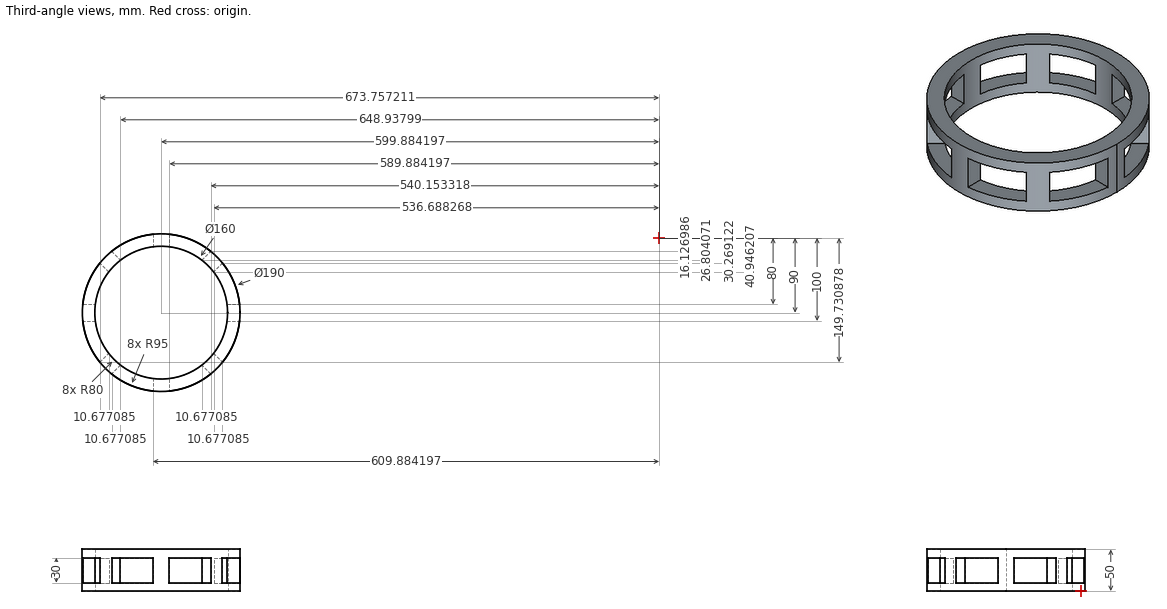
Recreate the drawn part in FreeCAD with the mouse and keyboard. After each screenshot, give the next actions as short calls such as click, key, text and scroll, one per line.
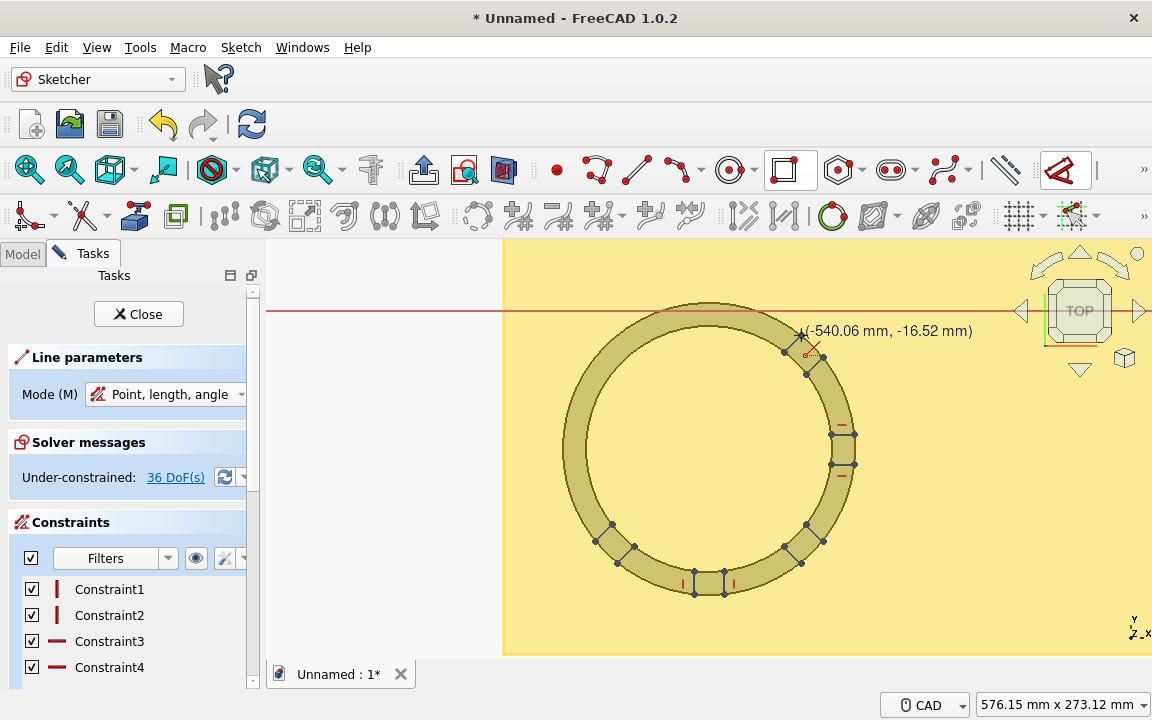
scroll(724, 304, up, 5)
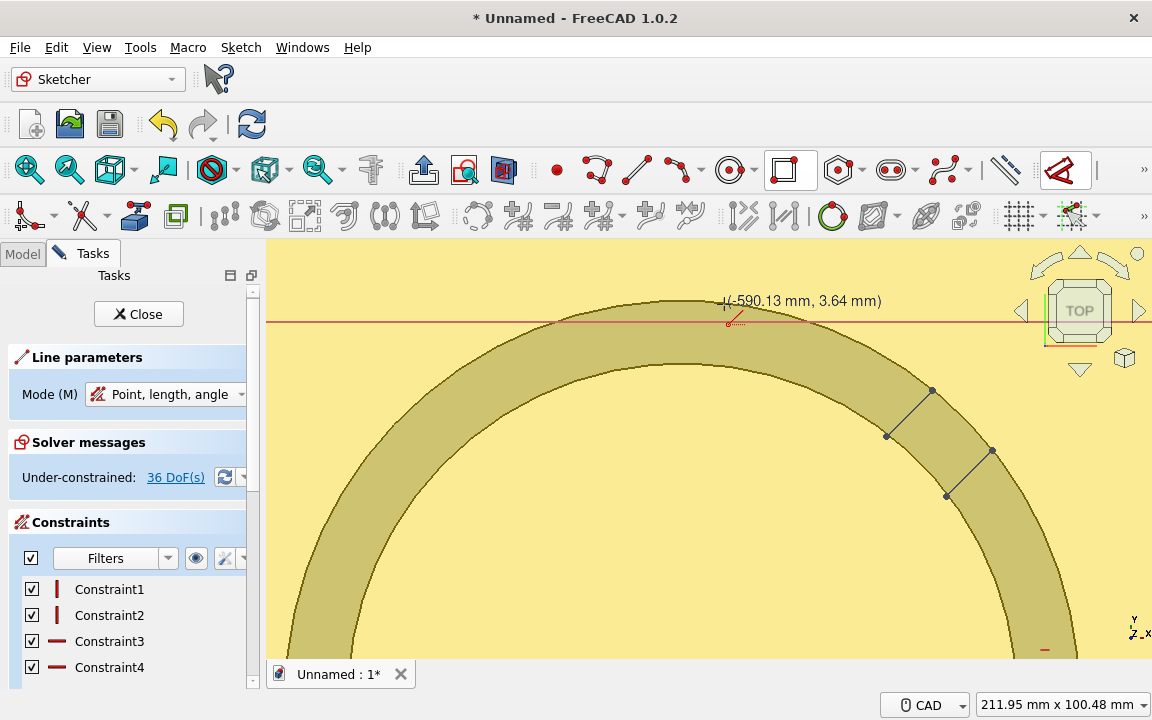
click(724, 303)
click(724, 366)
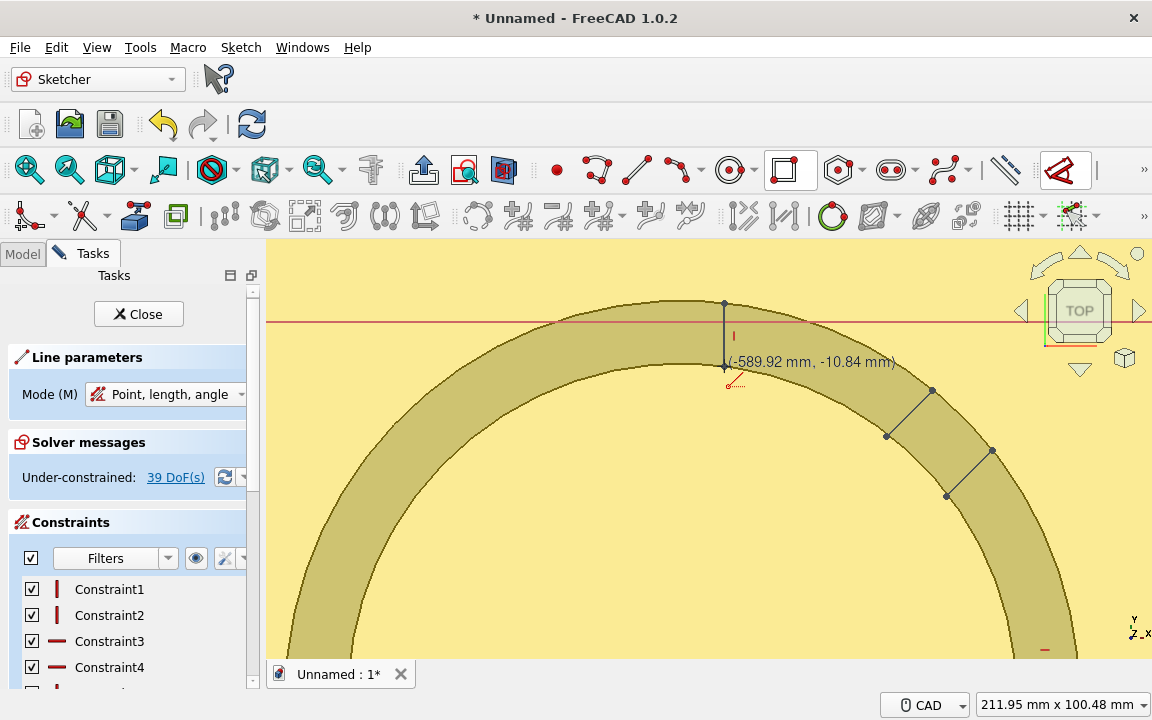
click(641, 366)
click(641, 303)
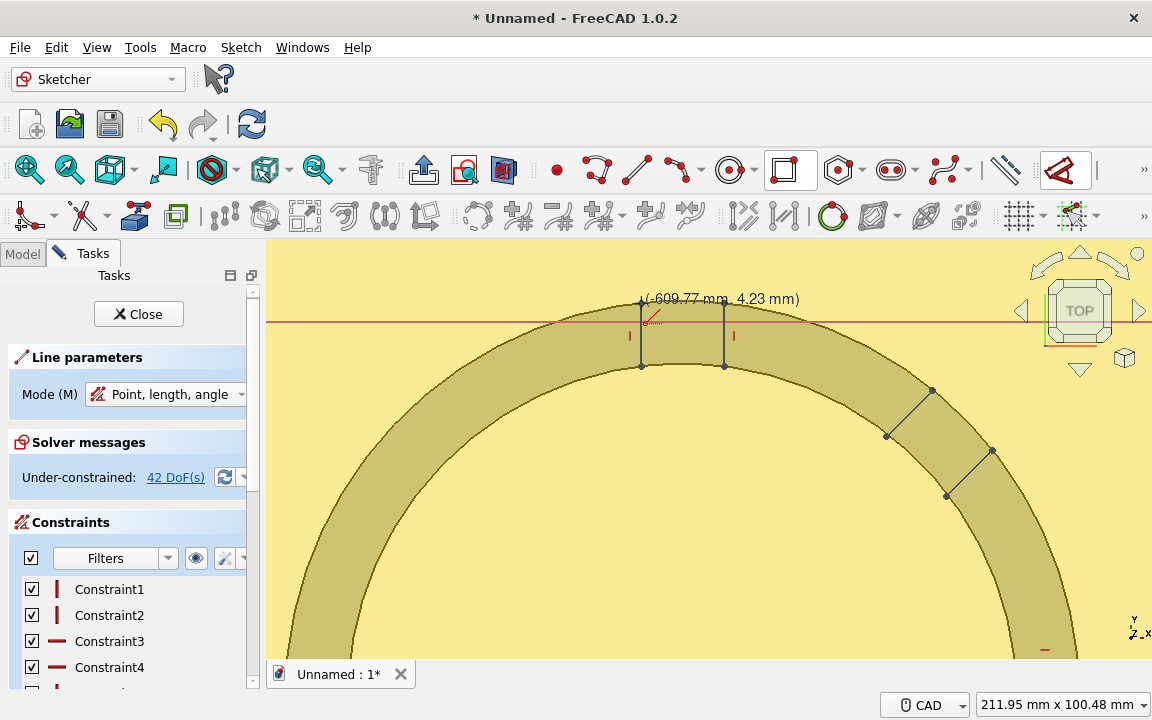
click(433, 389)
click(477, 434)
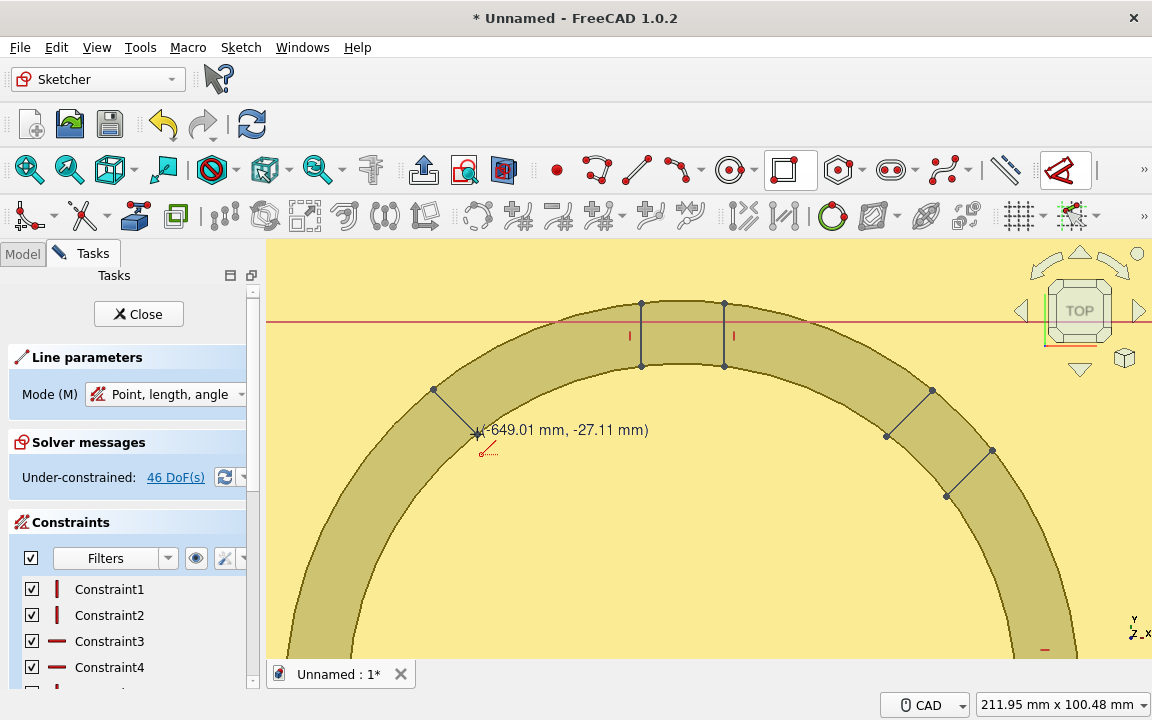
click(418, 493)
click(374, 448)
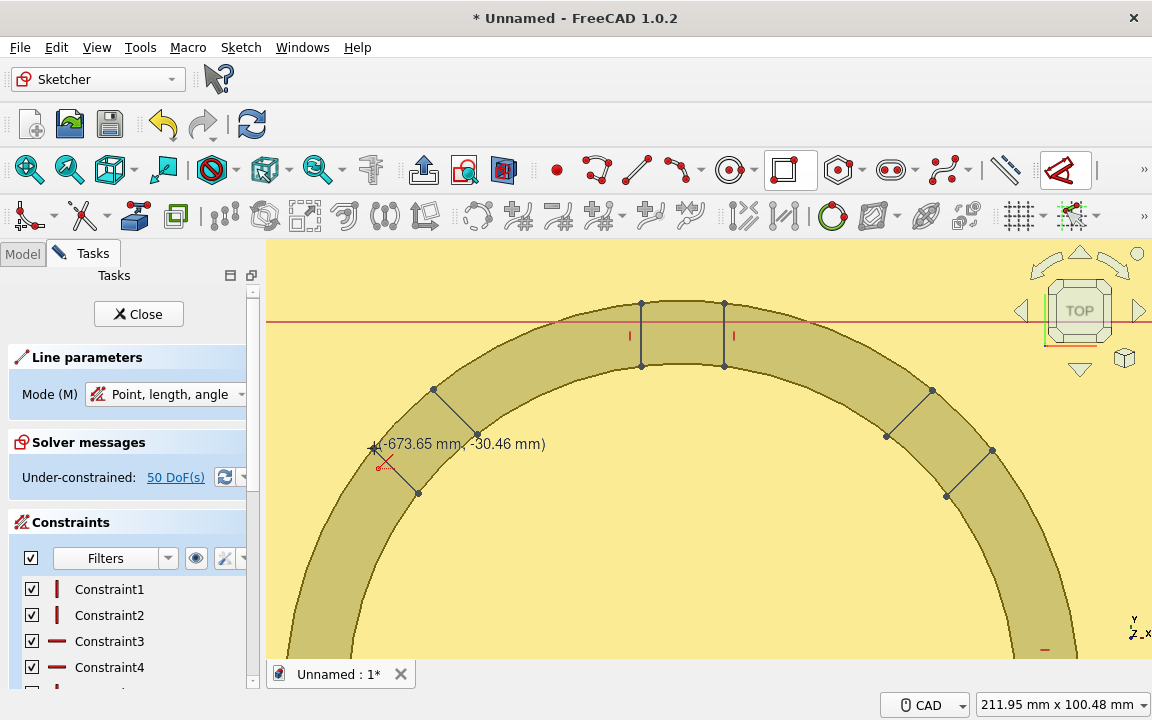
scroll(622, 342, down, 6)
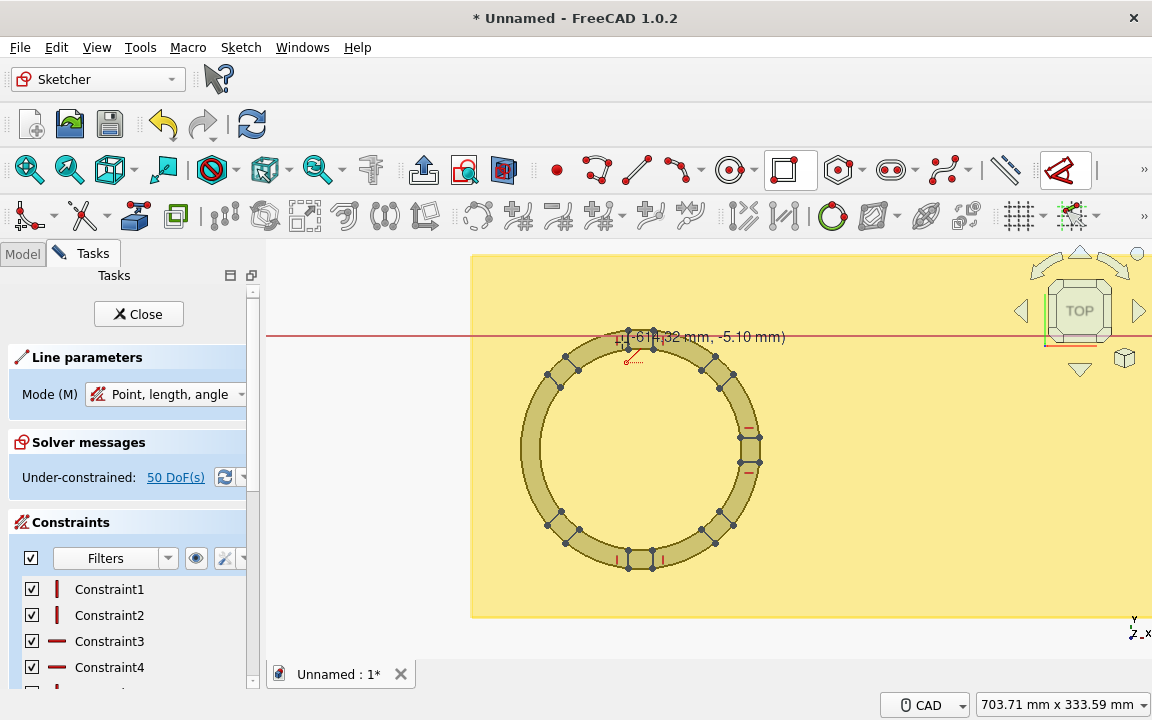
click(522, 437)
click(541, 437)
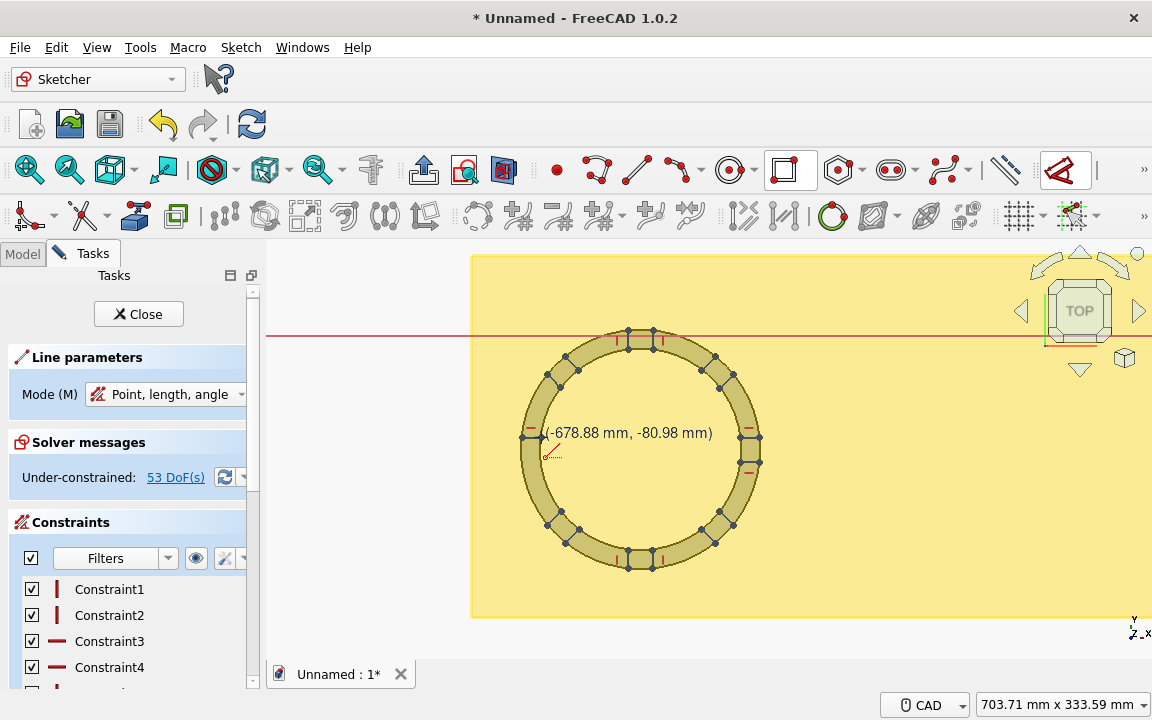
click(541, 462)
click(522, 462)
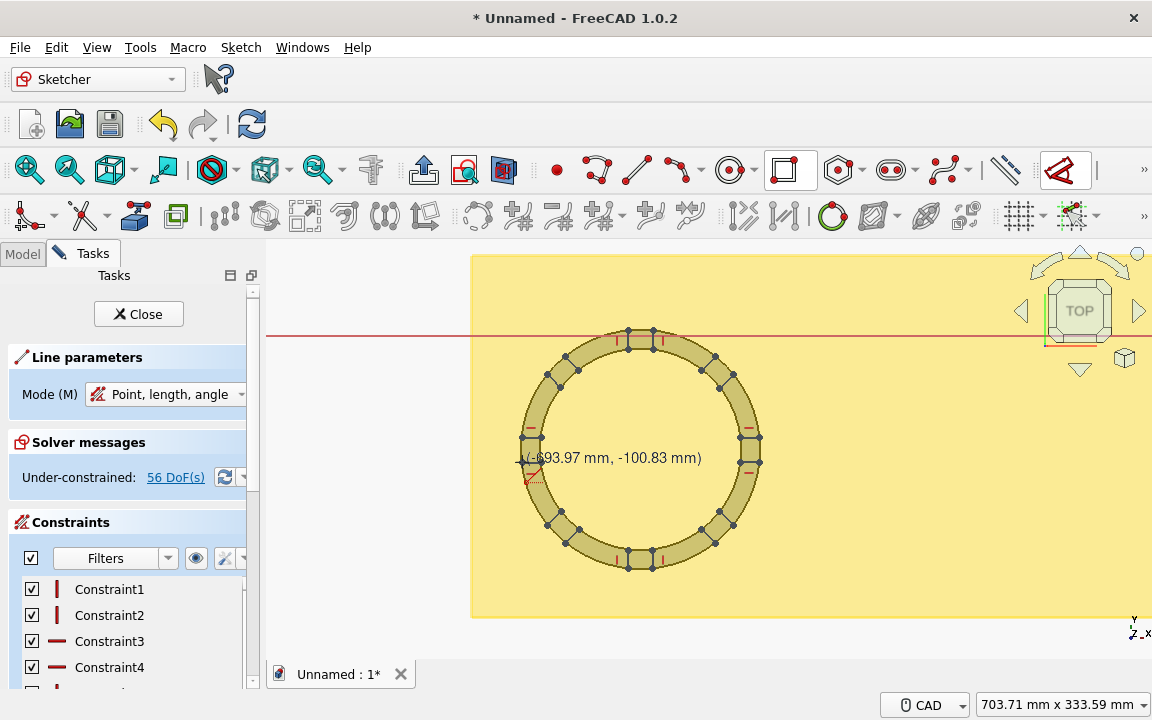
click(678, 170)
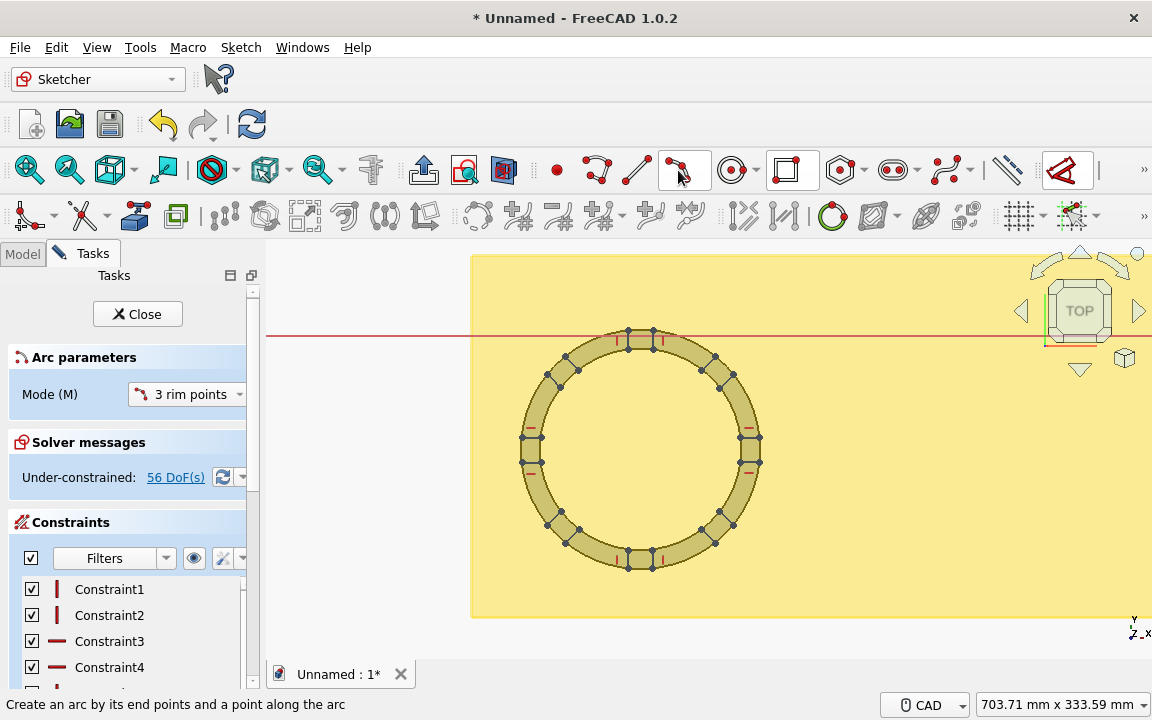
scroll(561, 511, up, 3)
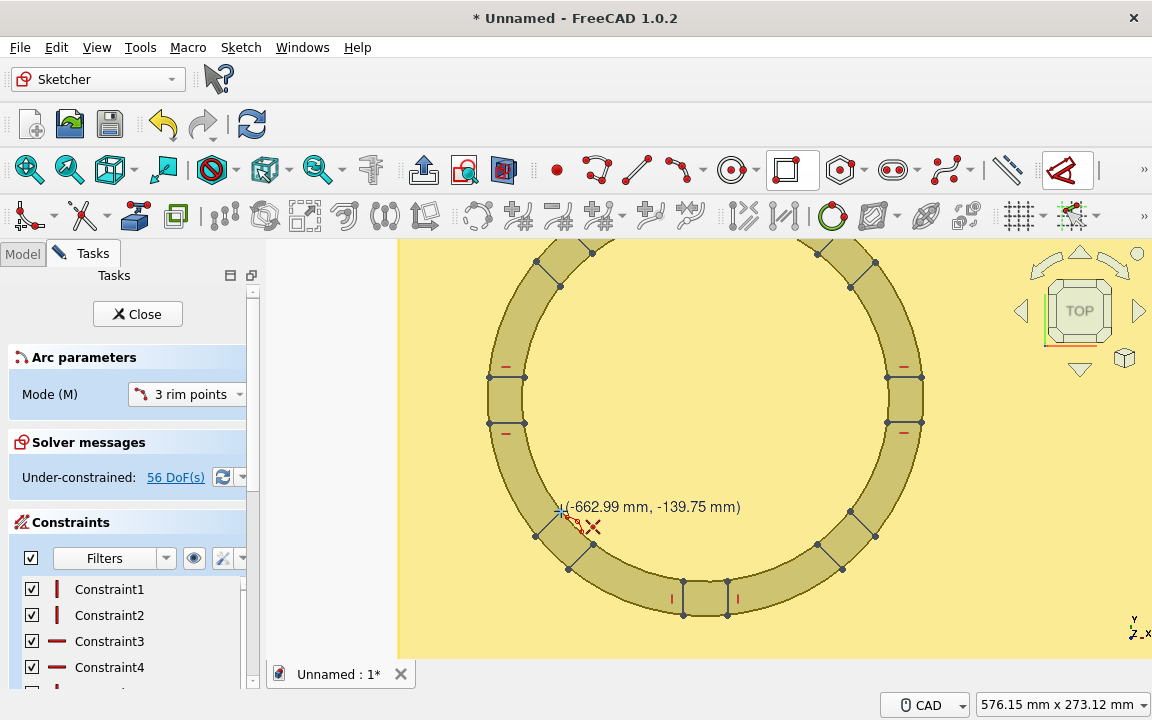
click(561, 512)
click(594, 544)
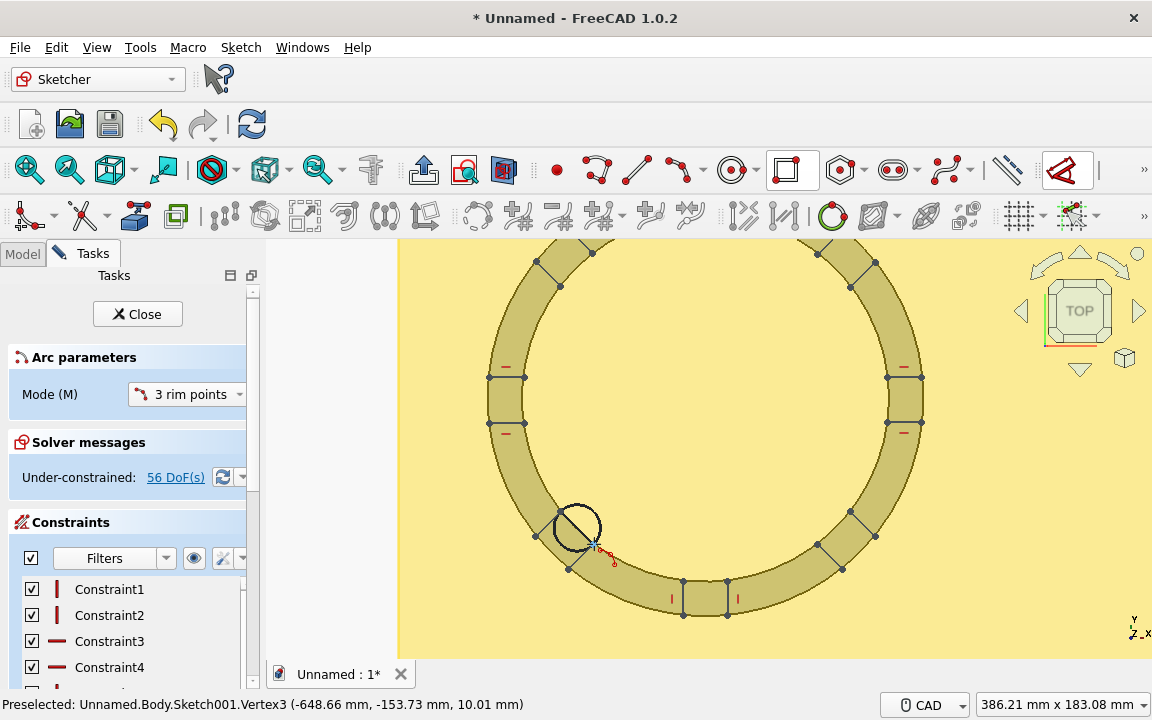
scroll(576, 528, up, 13)